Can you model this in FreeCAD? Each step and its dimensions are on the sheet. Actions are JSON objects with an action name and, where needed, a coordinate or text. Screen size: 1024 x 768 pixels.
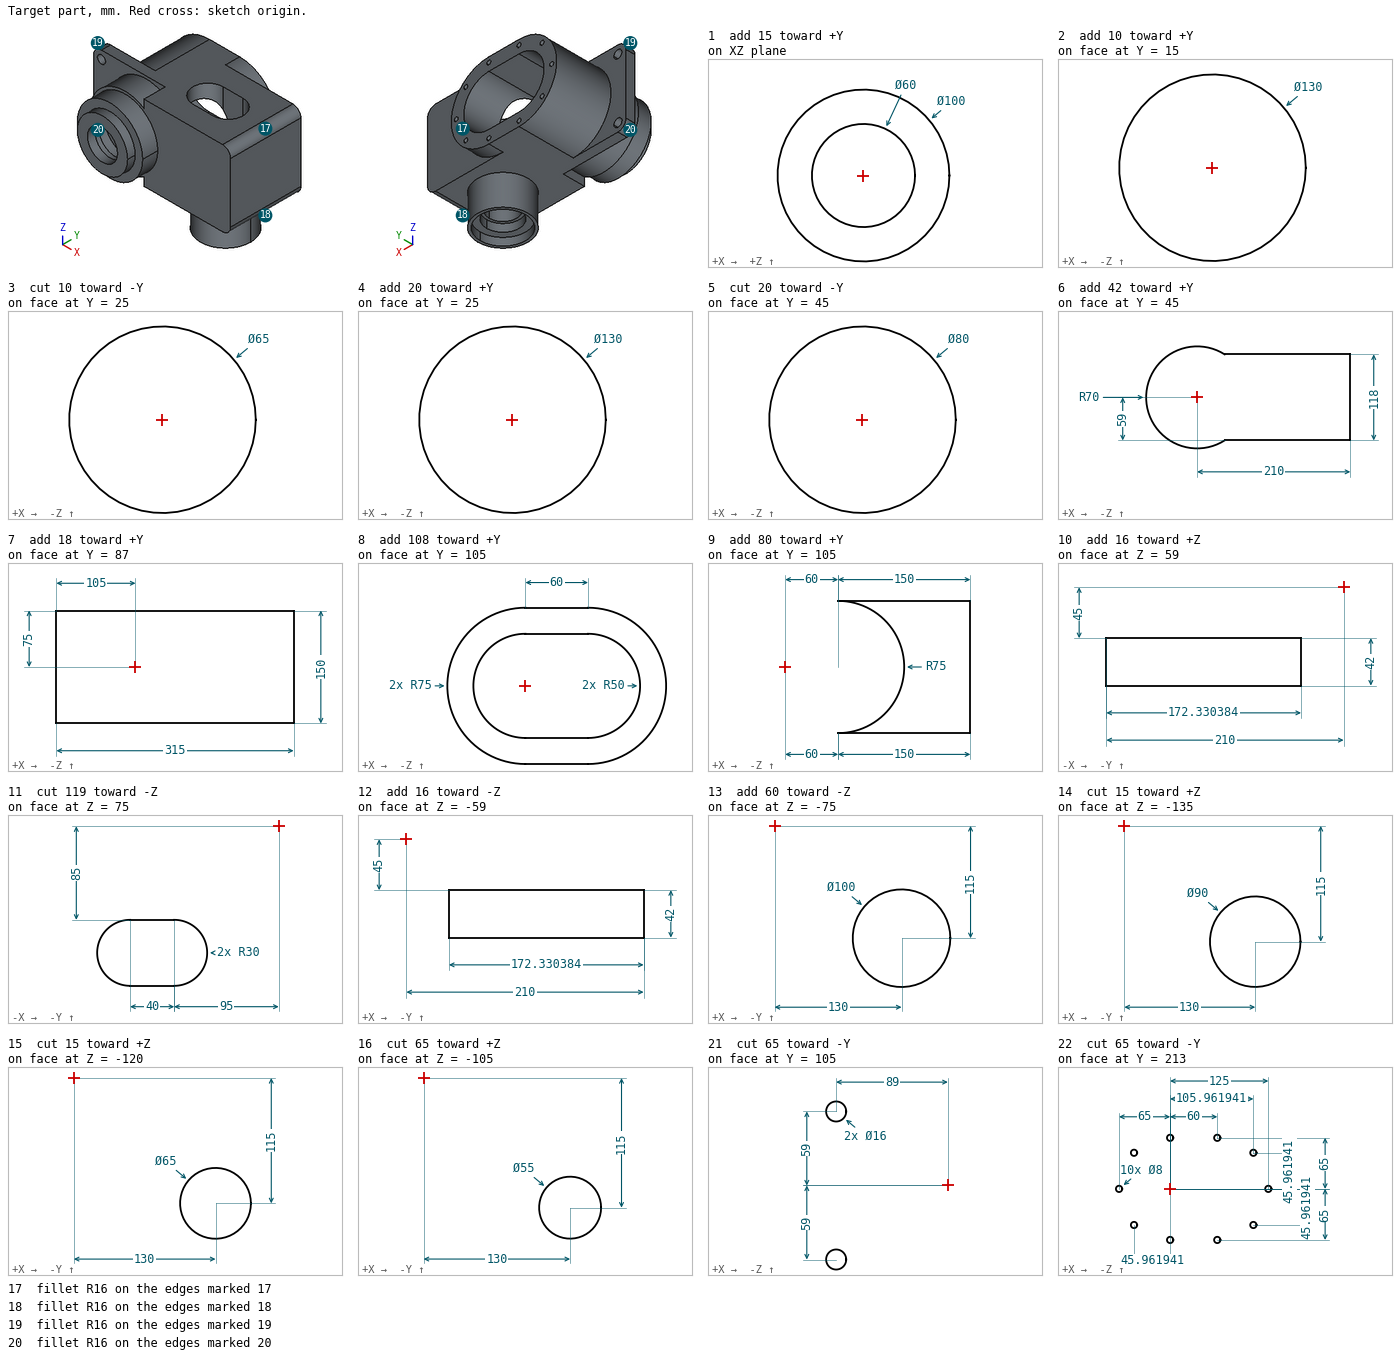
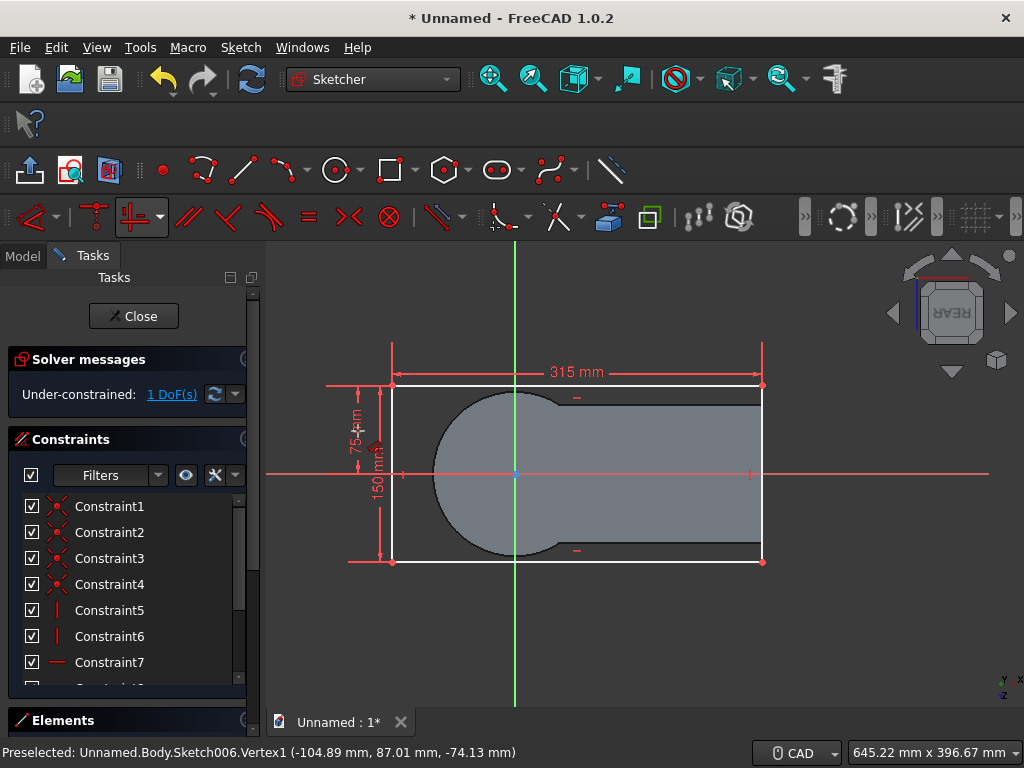
{"action": "left_click", "coordinate": [392, 386]}
{"action": "left_click", "coordinate": [454, 352]}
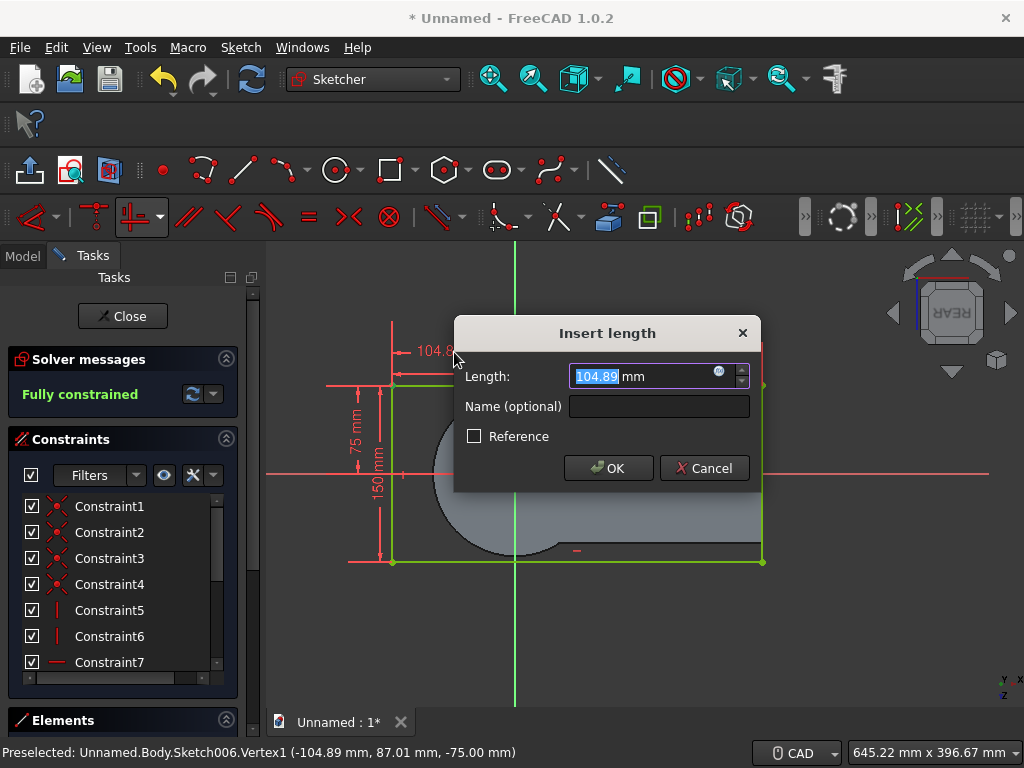
{"action": "type", "text": "105"}
{"action": "key", "text": "Return"}
{"action": "key", "text": "Escape"}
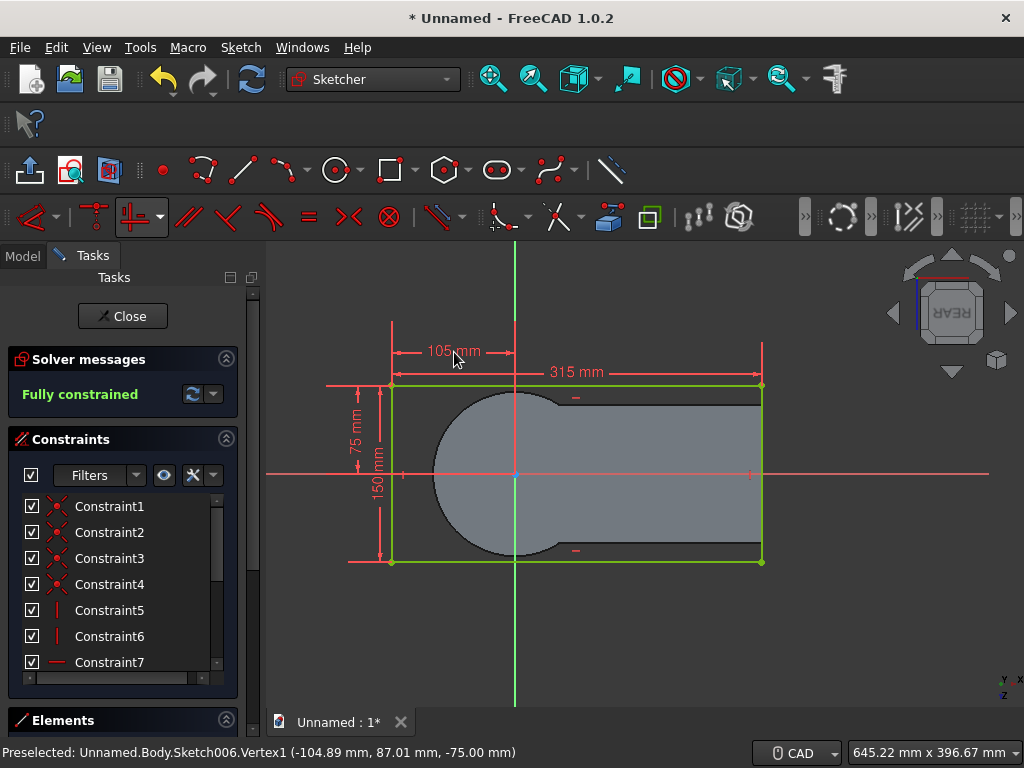
{"action": "left_click", "coordinate": [123, 316]}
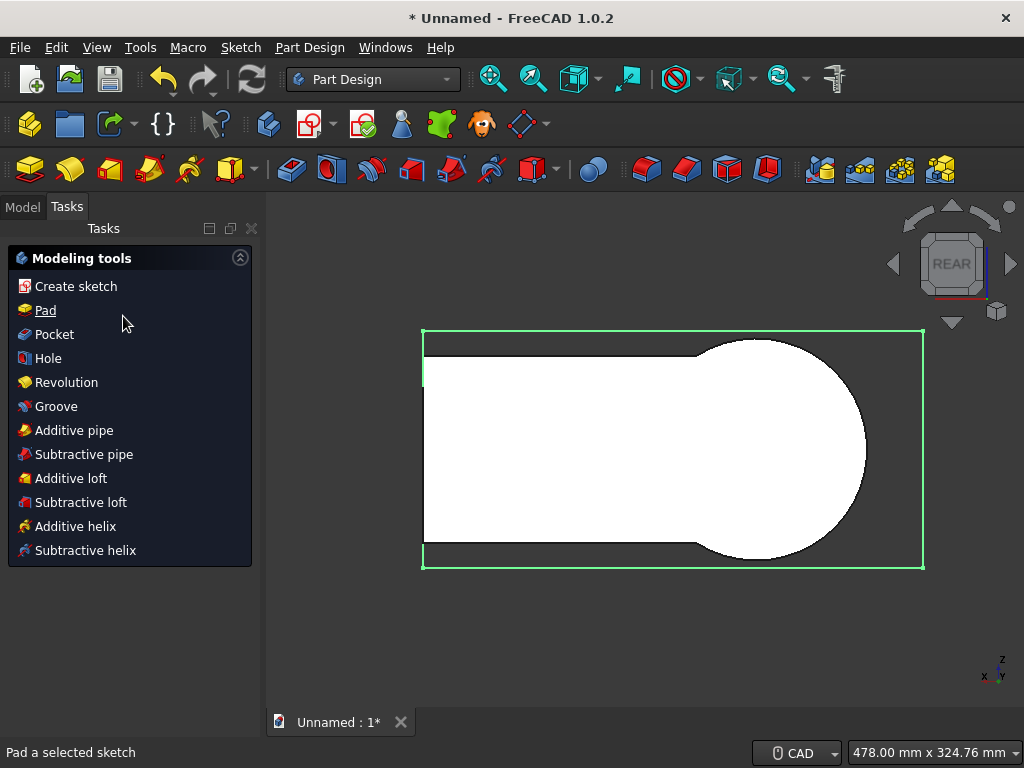
{"action": "left_click", "coordinate": [30, 170]}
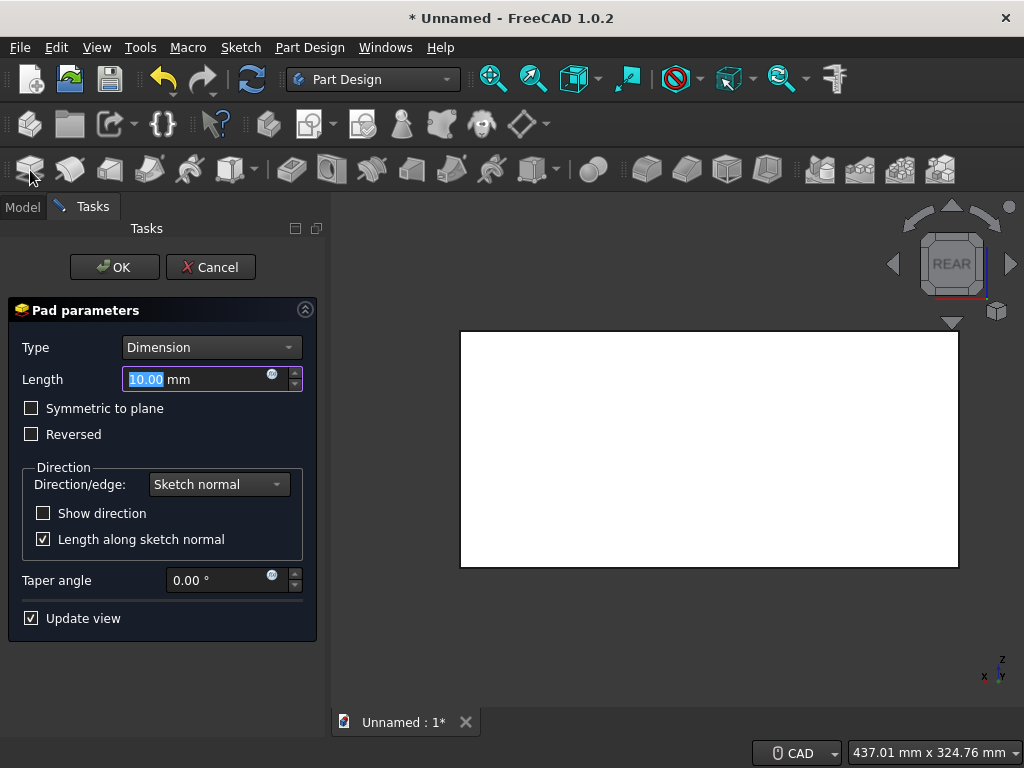
{"action": "type", "text": "18"}
{"action": "key", "text": "Tab"}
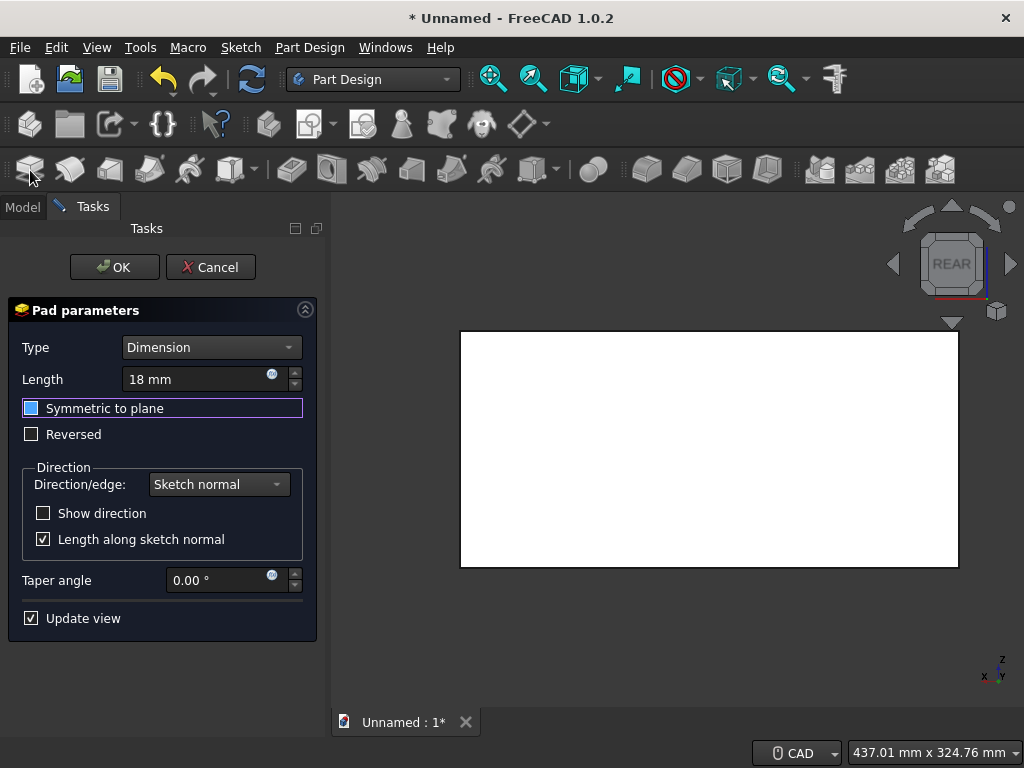
{"action": "left_click", "coordinate": [115, 267]}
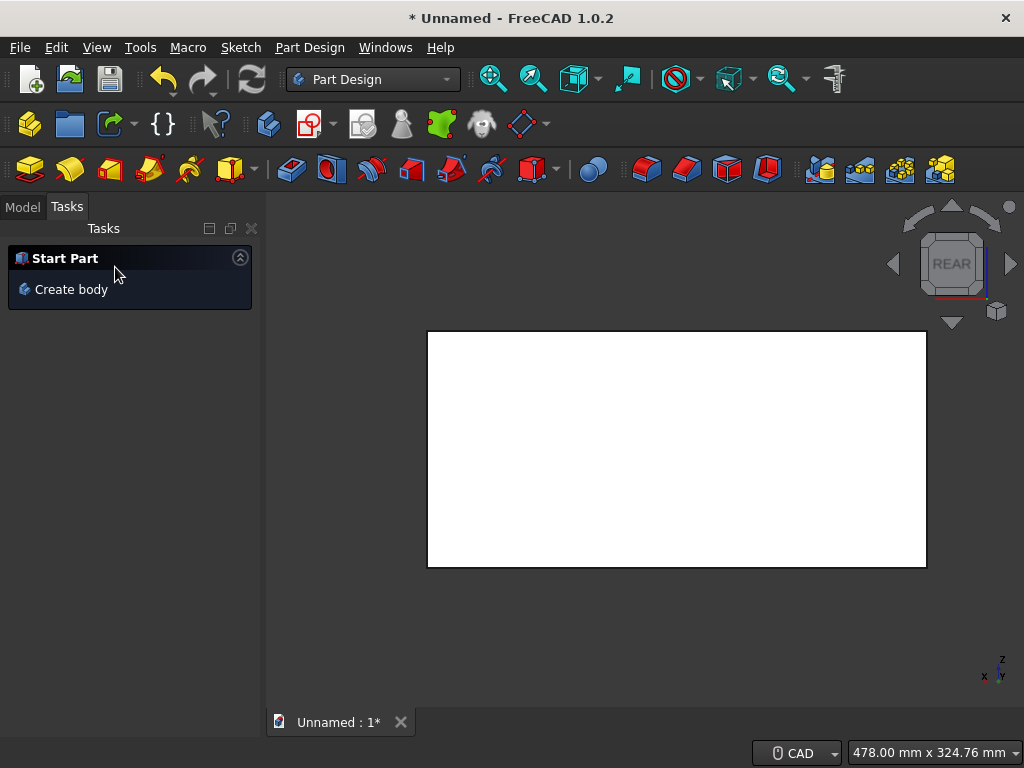
{"action": "left_click", "coordinate": [606, 448]}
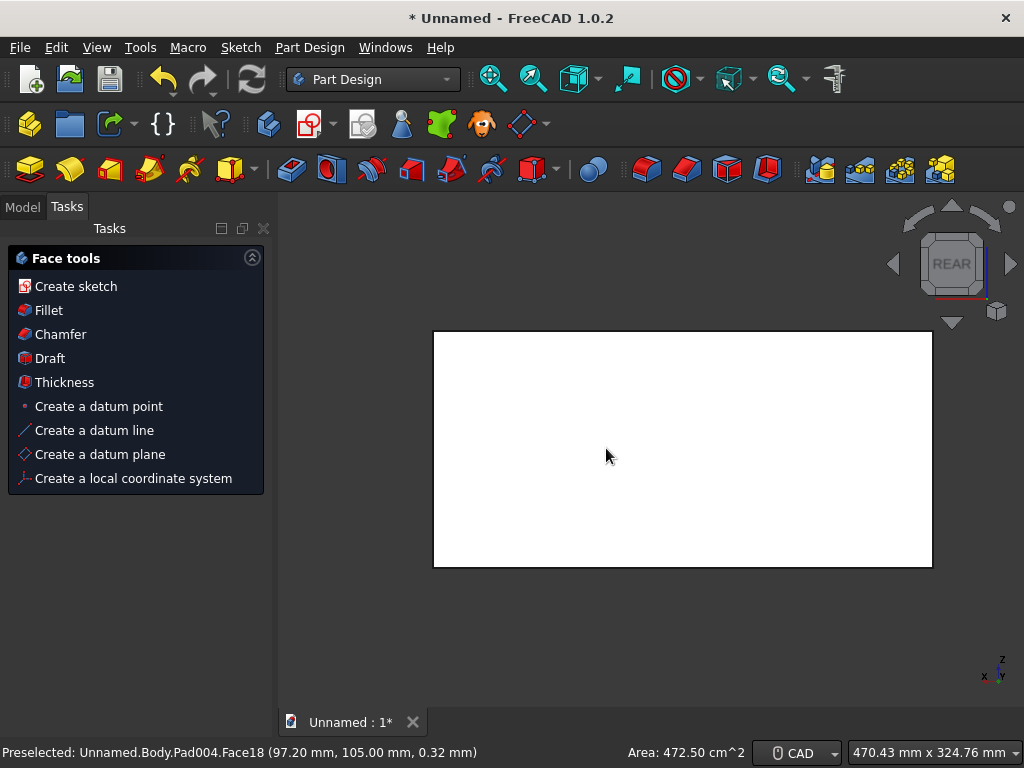
{"action": "left_click", "coordinate": [310, 124]}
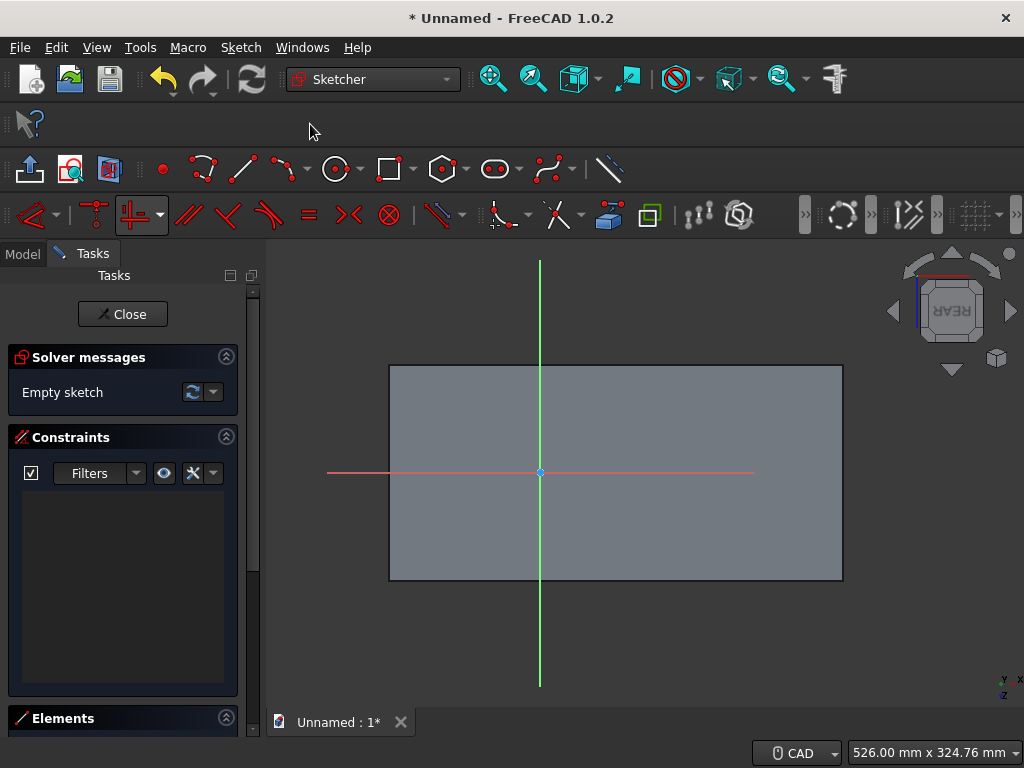
{"action": "left_click", "coordinate": [496, 170]}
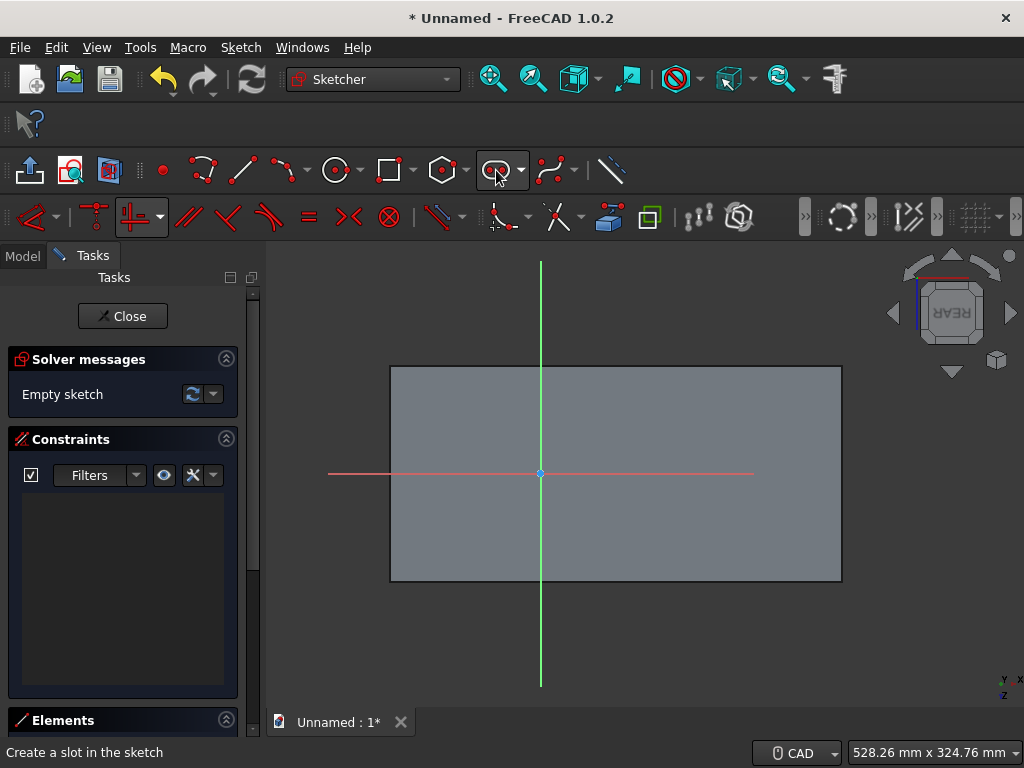
{"action": "left_click", "coordinate": [541, 474]}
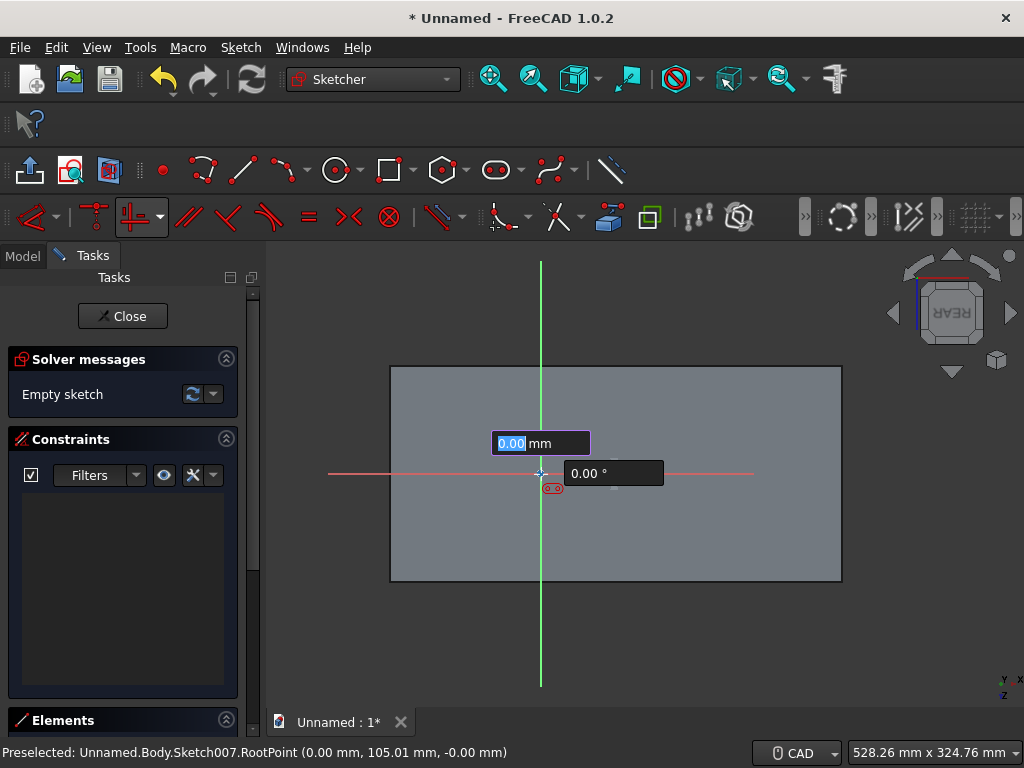
{"action": "left_click", "coordinate": [627, 465]}